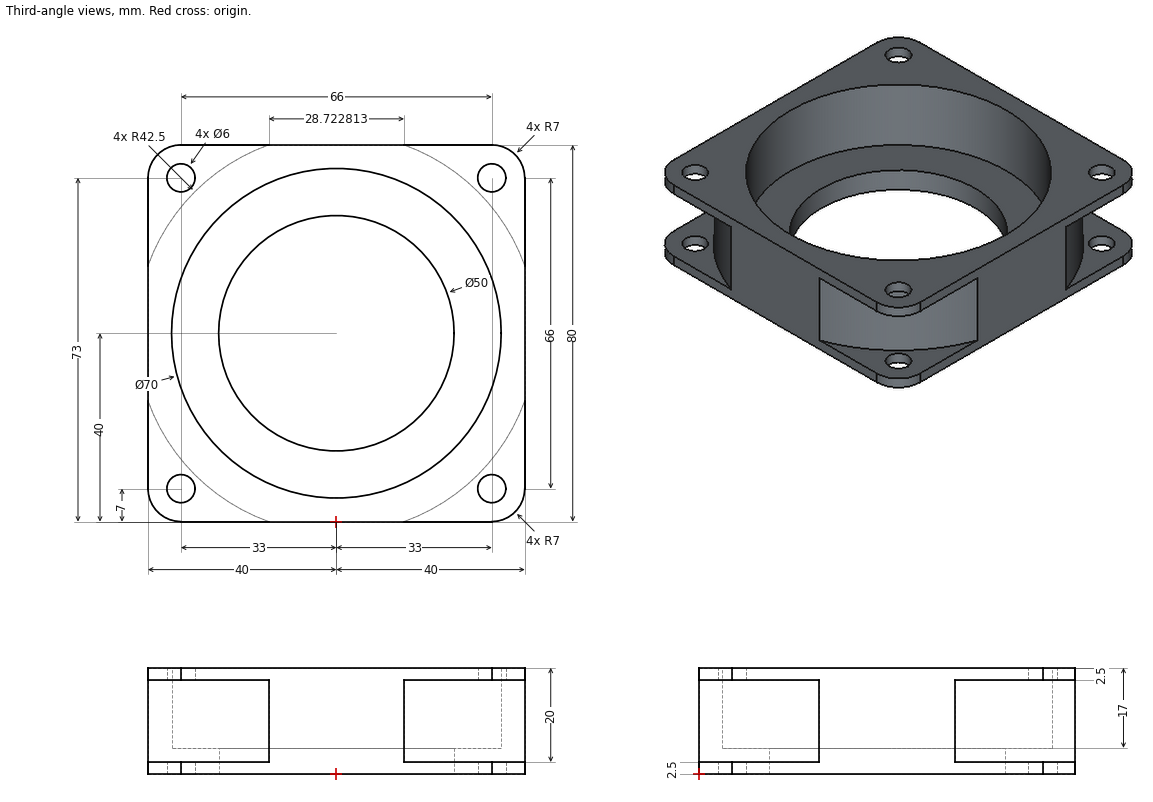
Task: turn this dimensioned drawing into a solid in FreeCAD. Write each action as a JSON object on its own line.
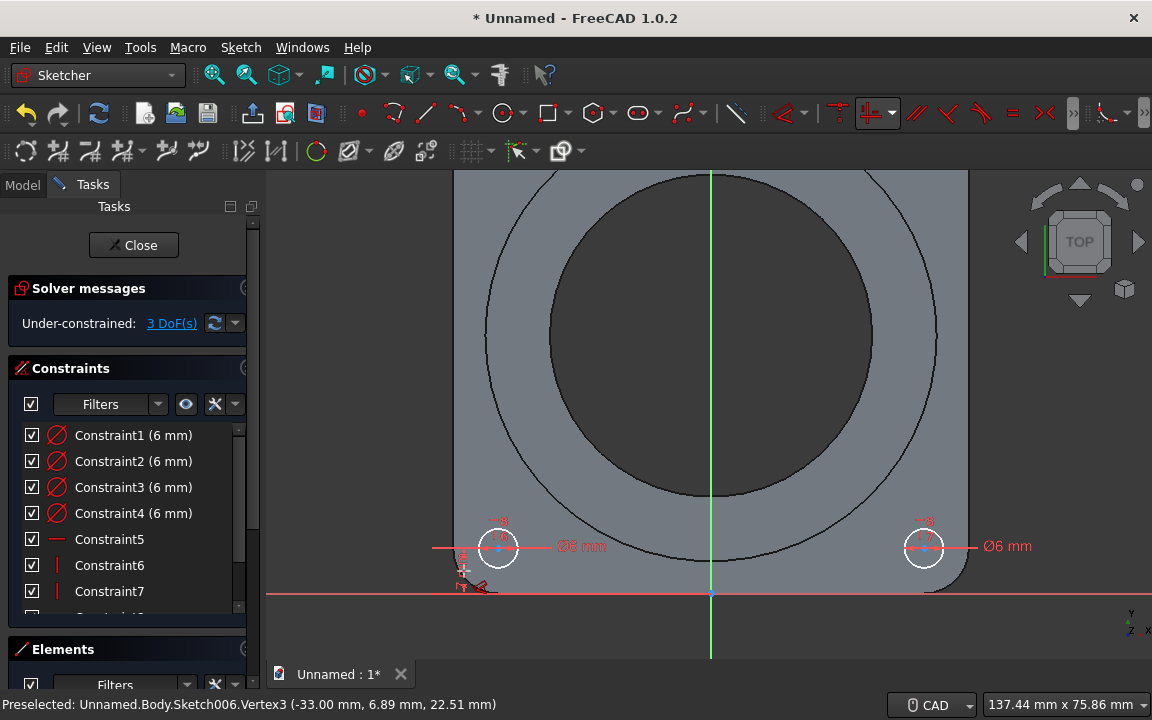
{"action": "scroll", "coordinate": [497, 549], "scroll_direction": "down", "scroll_amount": 2}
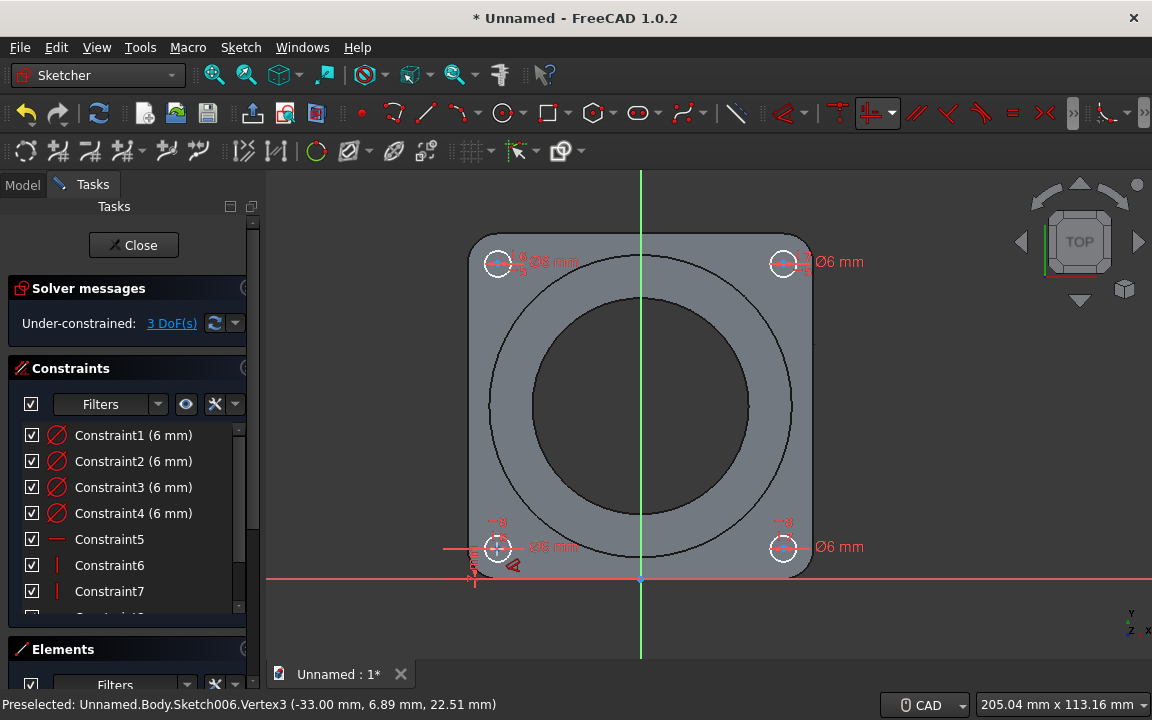
{"action": "left_click", "coordinate": [498, 264]}
{"action": "left_click", "coordinate": [569, 613]}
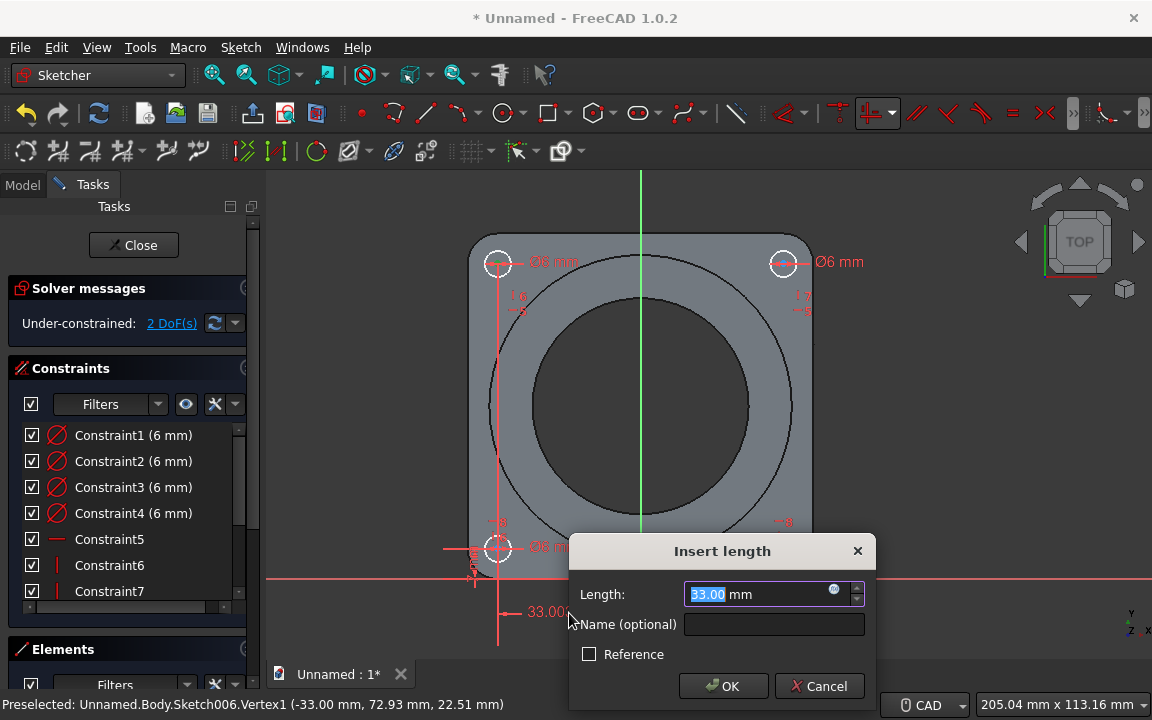
{"action": "type", "text": "33"}
{"action": "key", "text": "Return"}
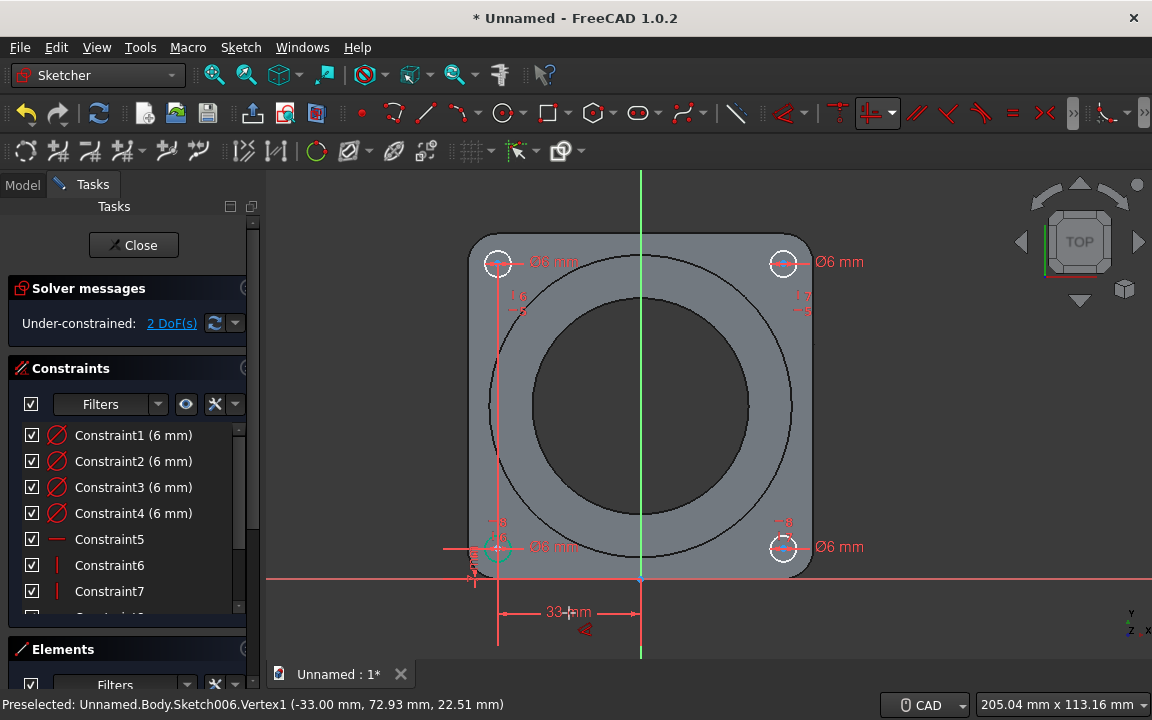
{"action": "left_click", "coordinate": [498, 264]}
{"action": "left_click", "coordinate": [464, 422]}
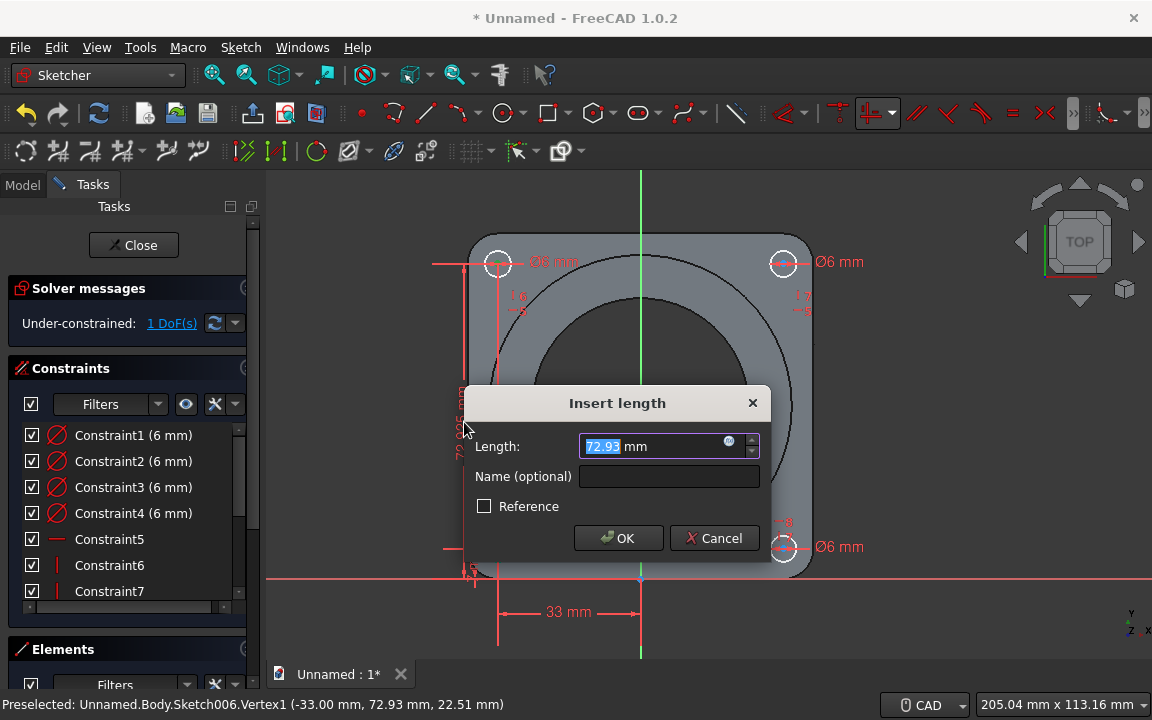
{"action": "type", "text": "73"}
{"action": "key", "text": "Return"}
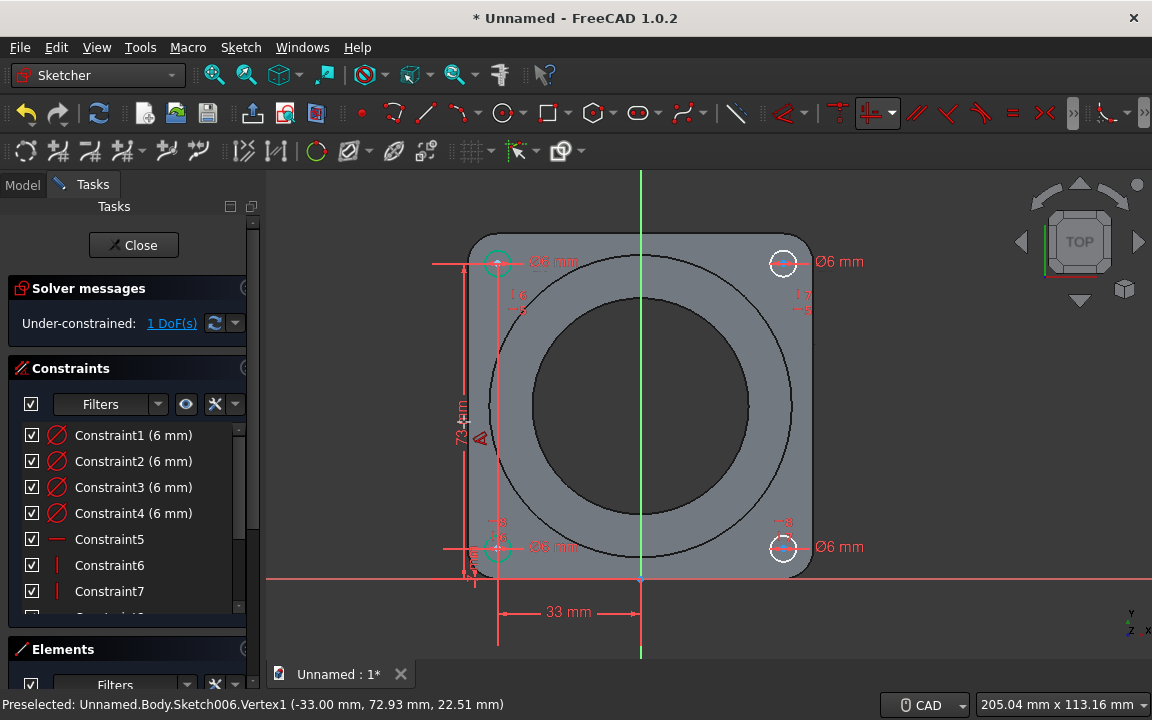
{"action": "left_click", "coordinate": [783, 264]}
{"action": "left_click", "coordinate": [712, 613]}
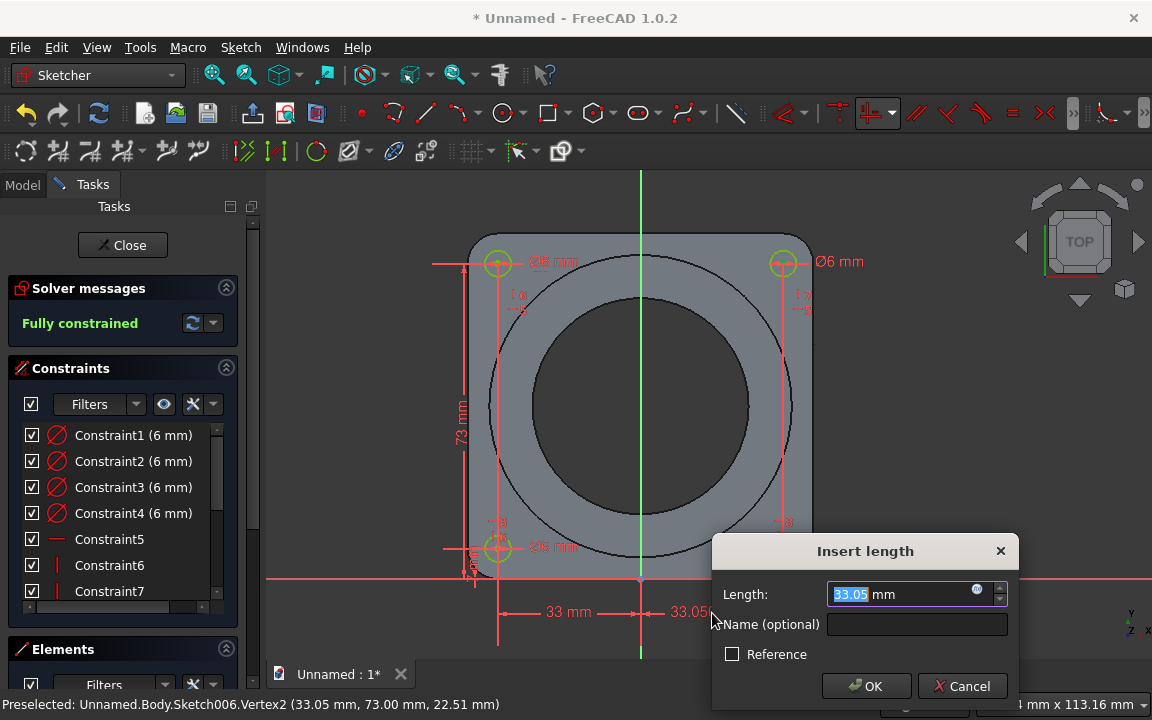
{"action": "type", "text": "33"}
{"action": "key", "text": "Return"}
{"action": "key", "text": "Escape"}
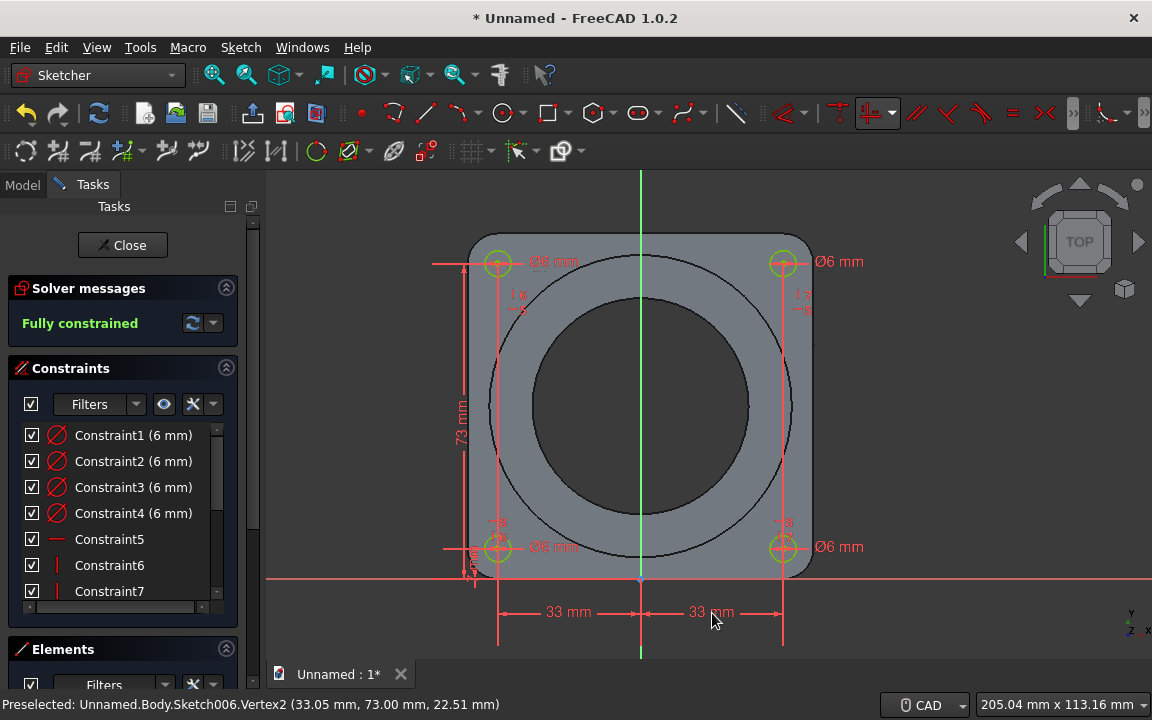
{"action": "left_click", "coordinate": [123, 245]}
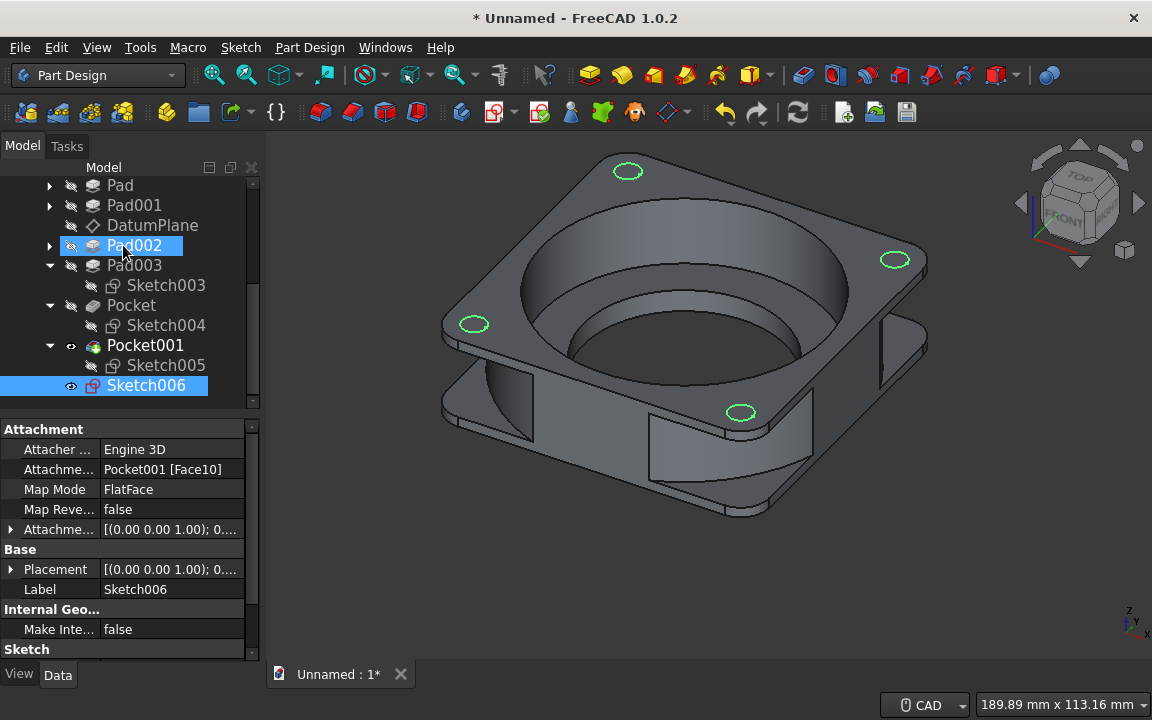
{"action": "left_click", "coordinate": [804, 76]}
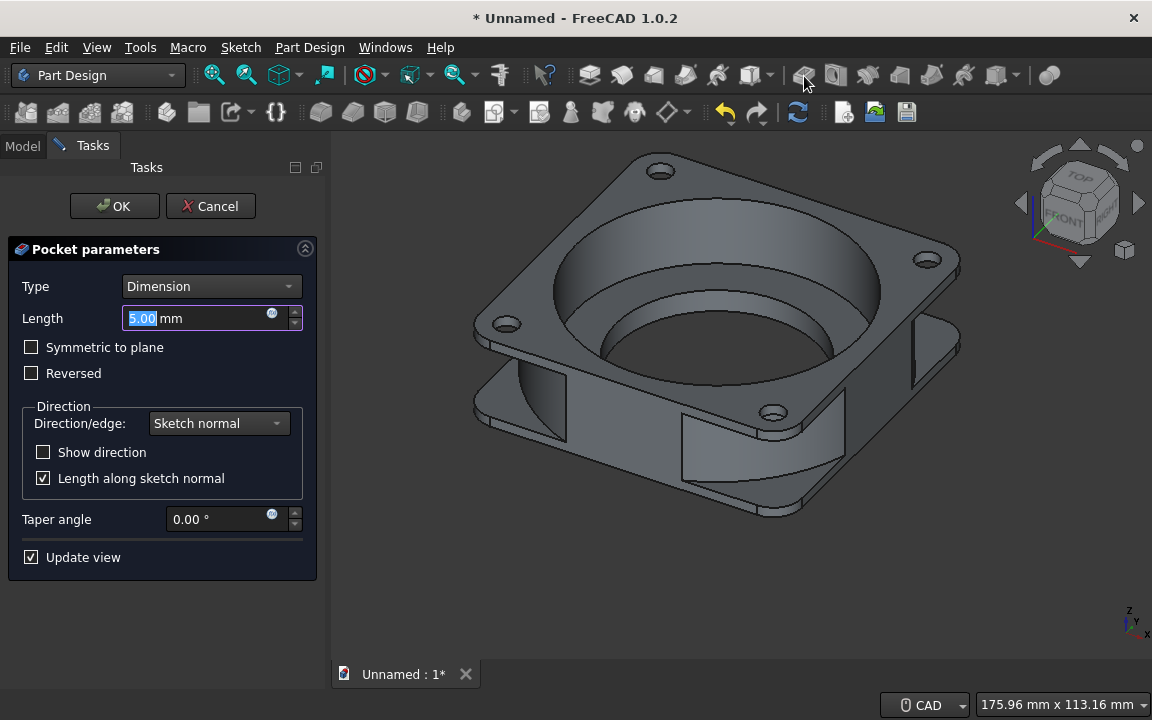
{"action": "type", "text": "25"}
{"action": "key", "text": "Tab"}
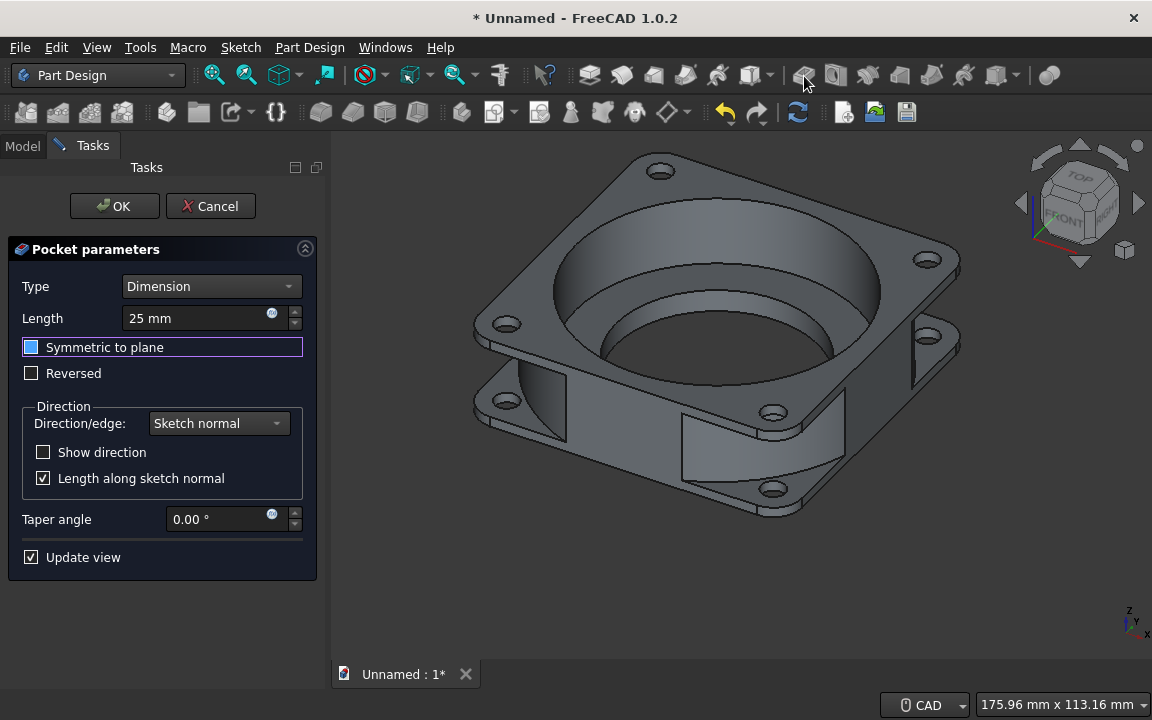
{"action": "left_click", "coordinate": [115, 206]}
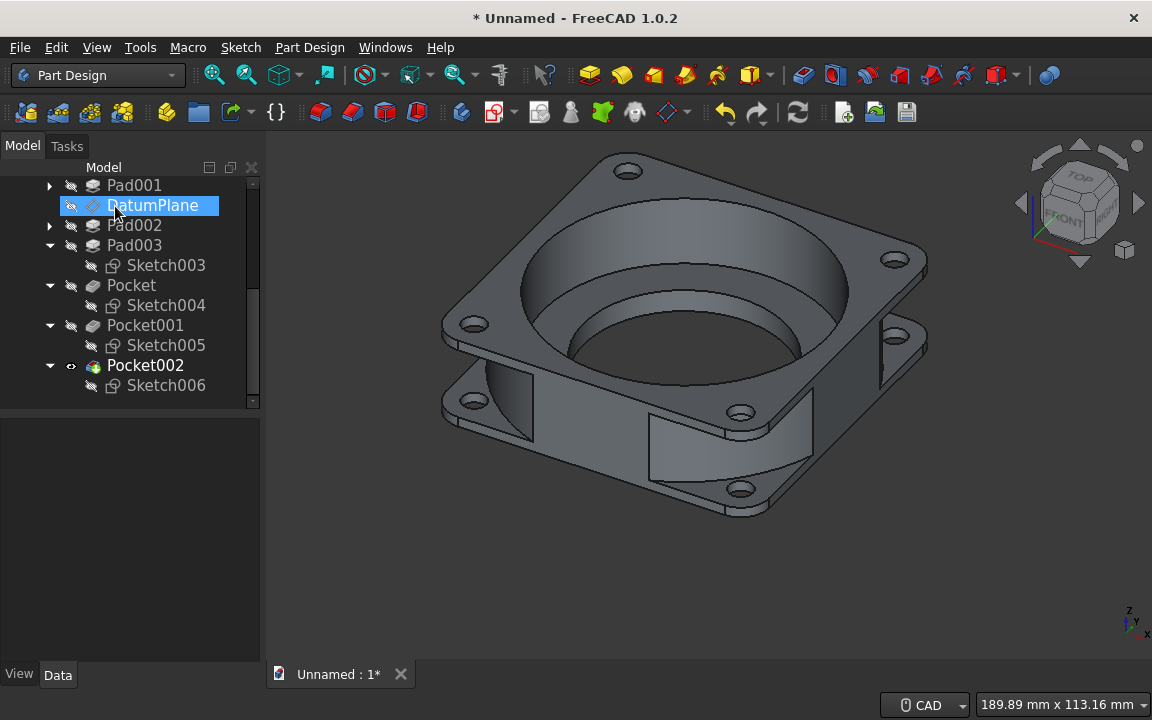
{"action": "key", "text": "0"}